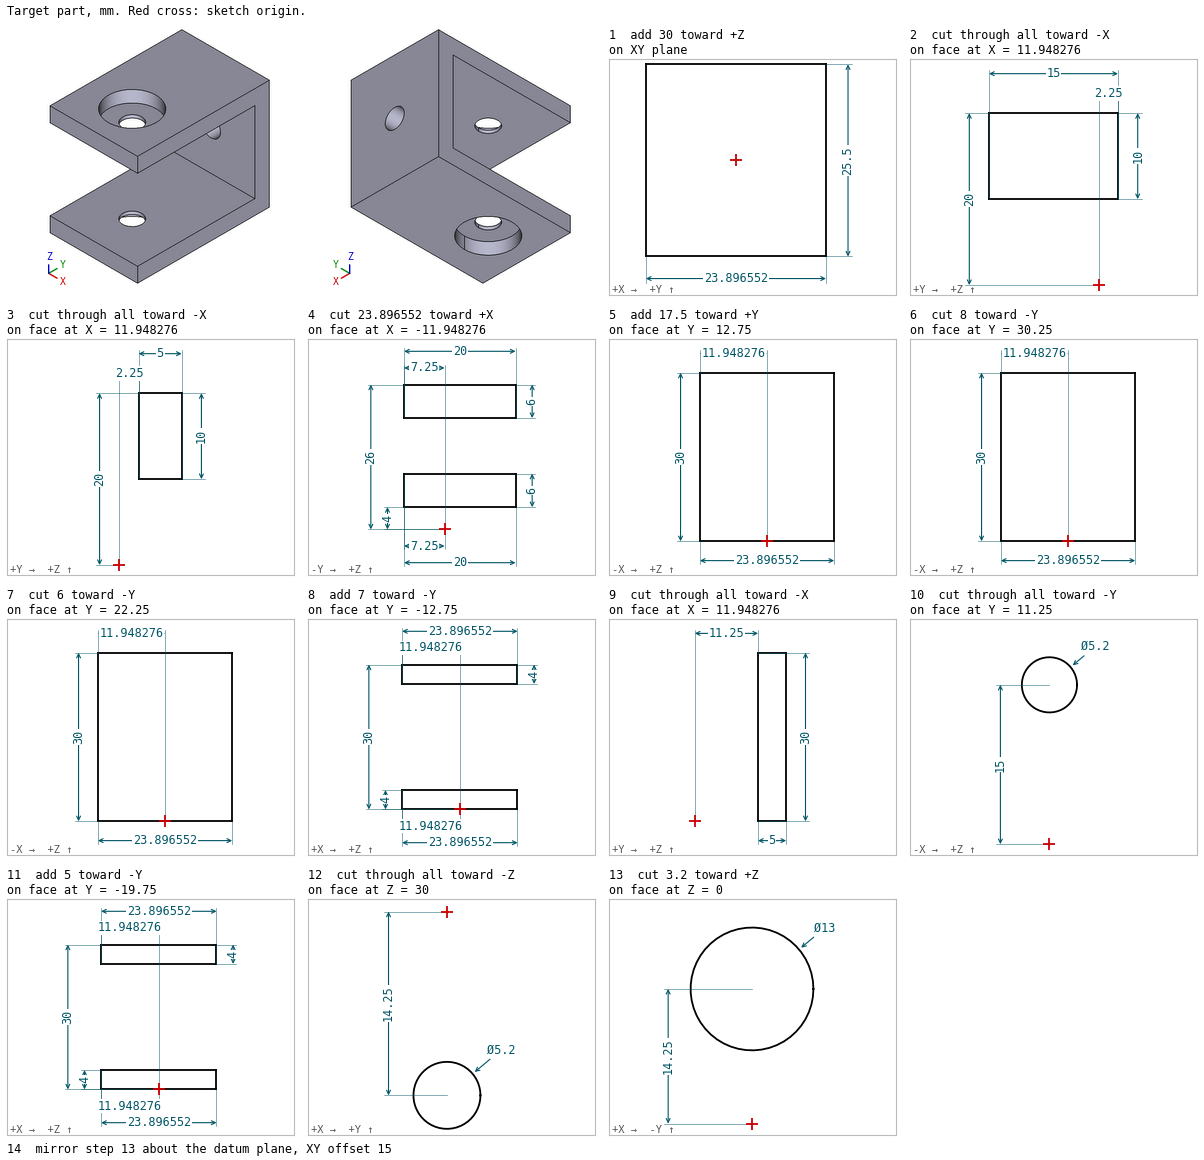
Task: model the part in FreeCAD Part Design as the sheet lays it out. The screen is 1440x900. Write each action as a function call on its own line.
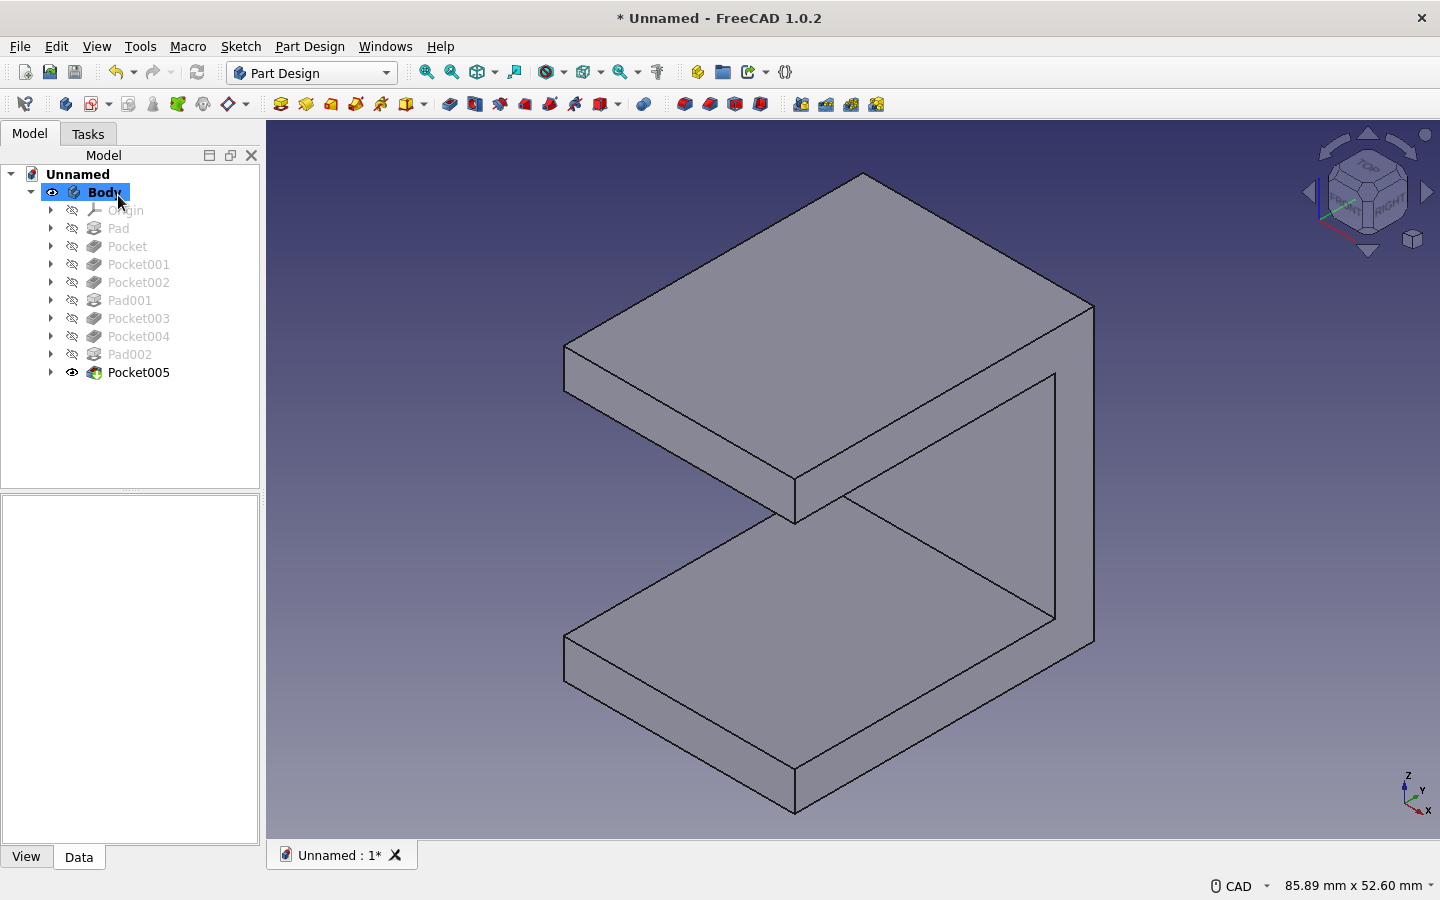
key(4)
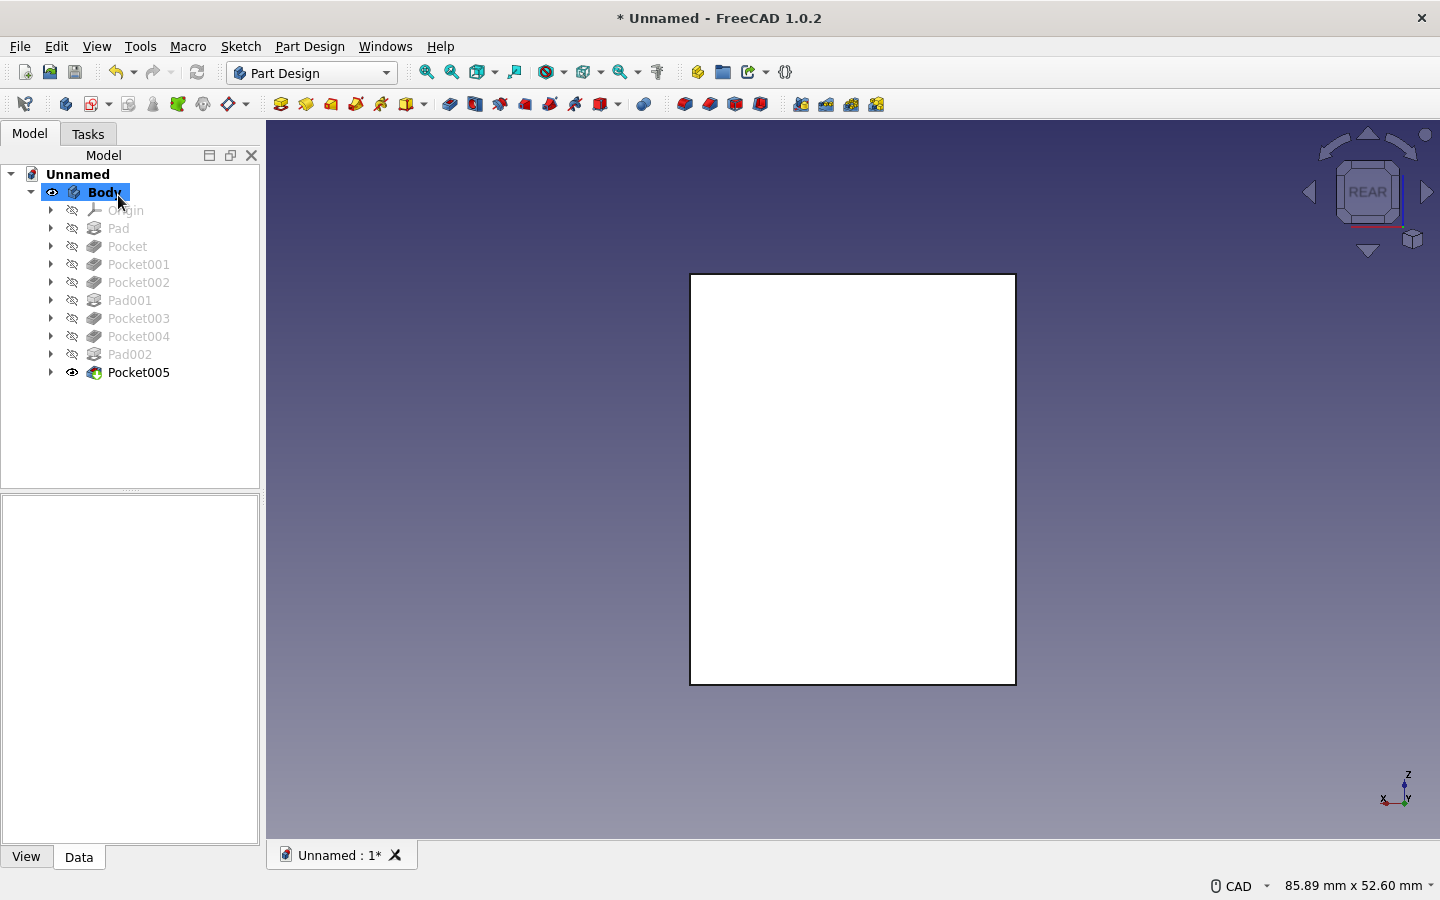
click(853, 479)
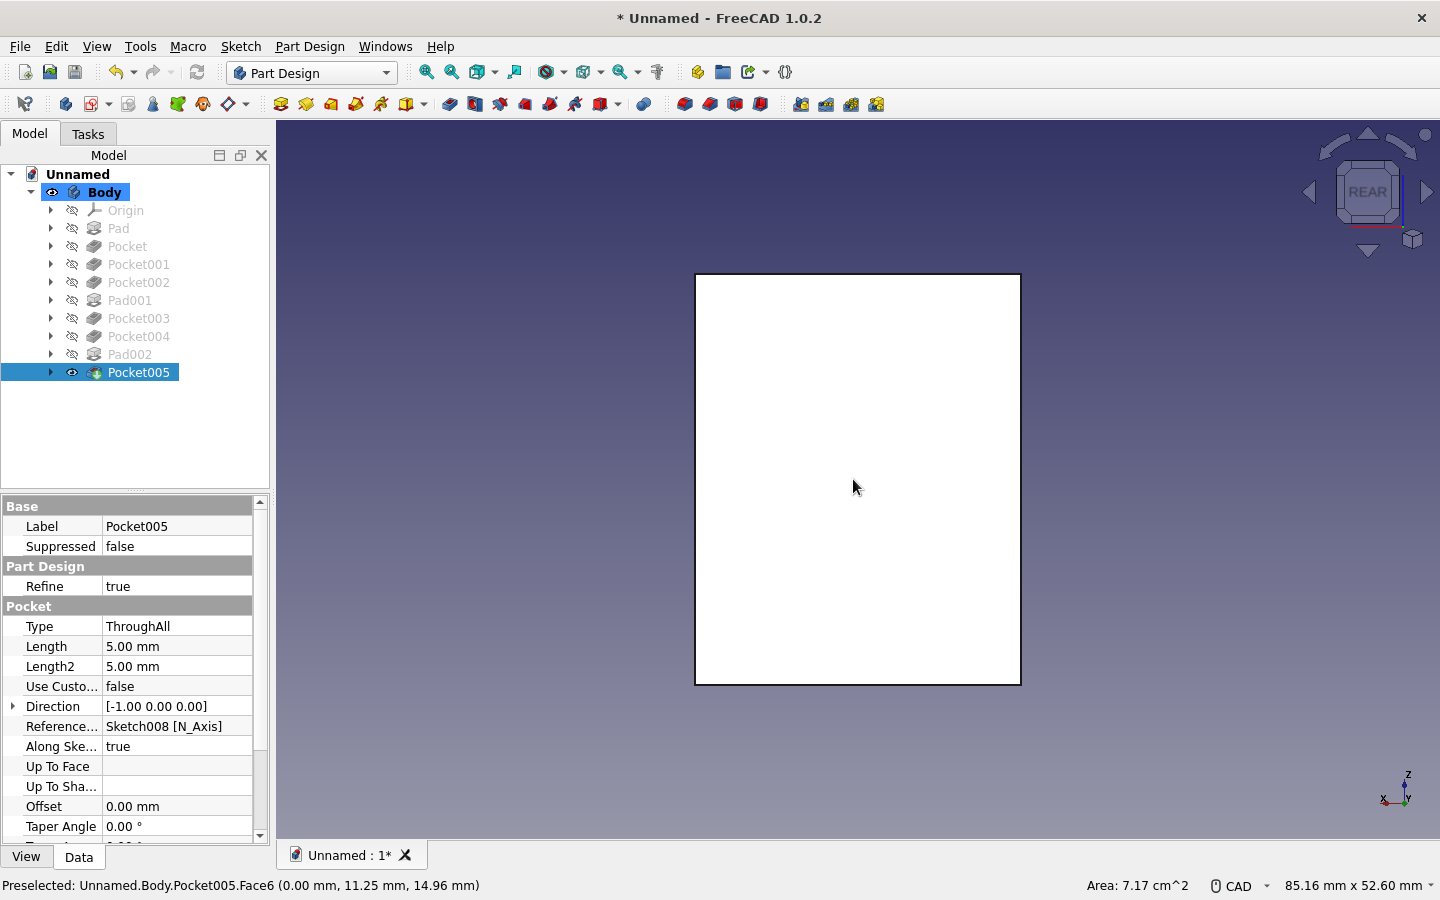
click(90, 104)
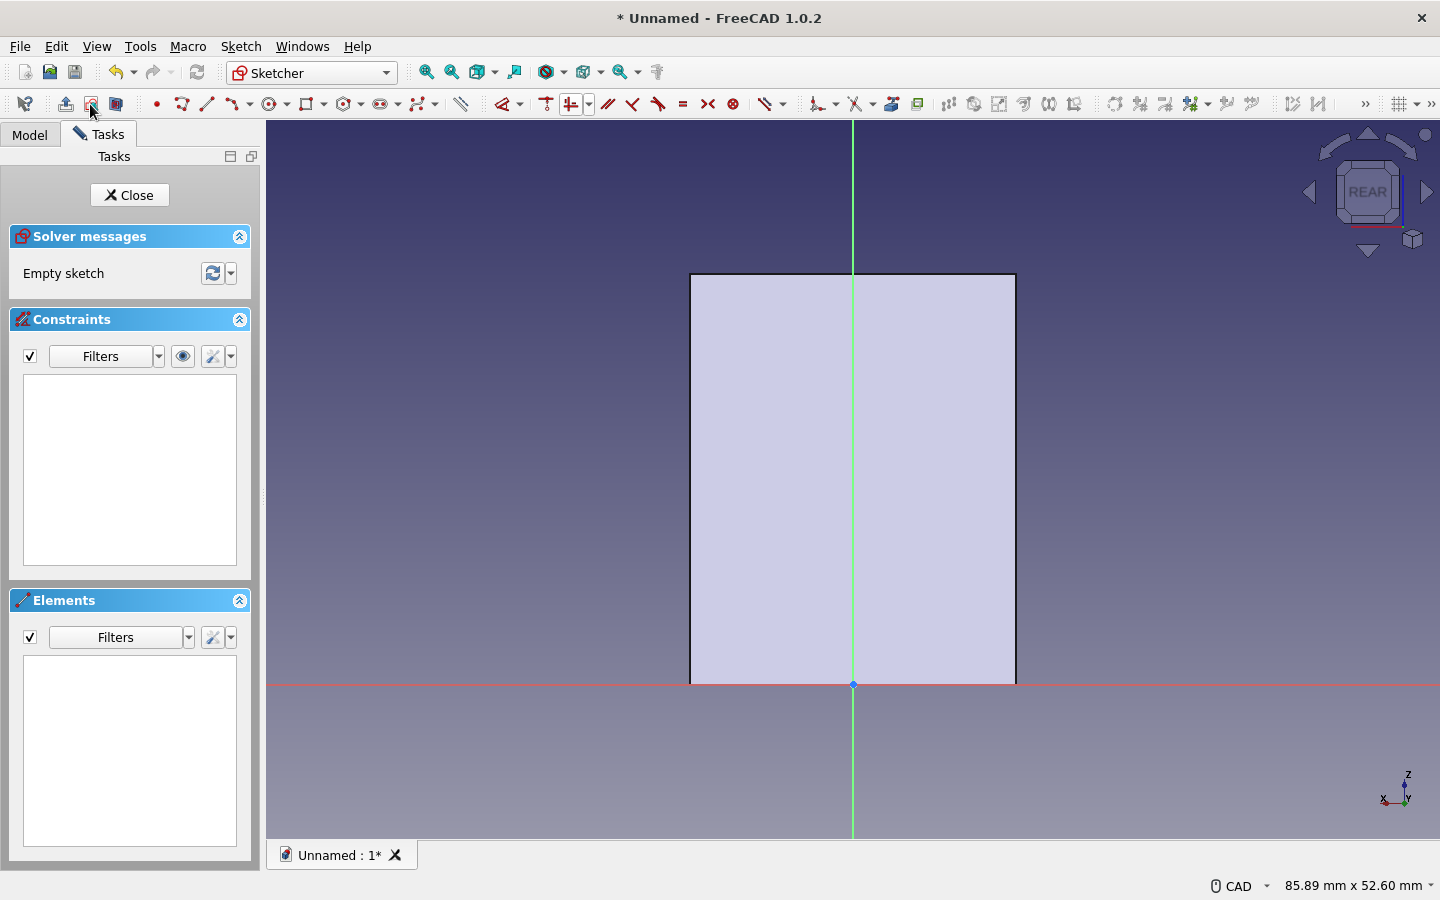
scroll(867, 480, up, 9)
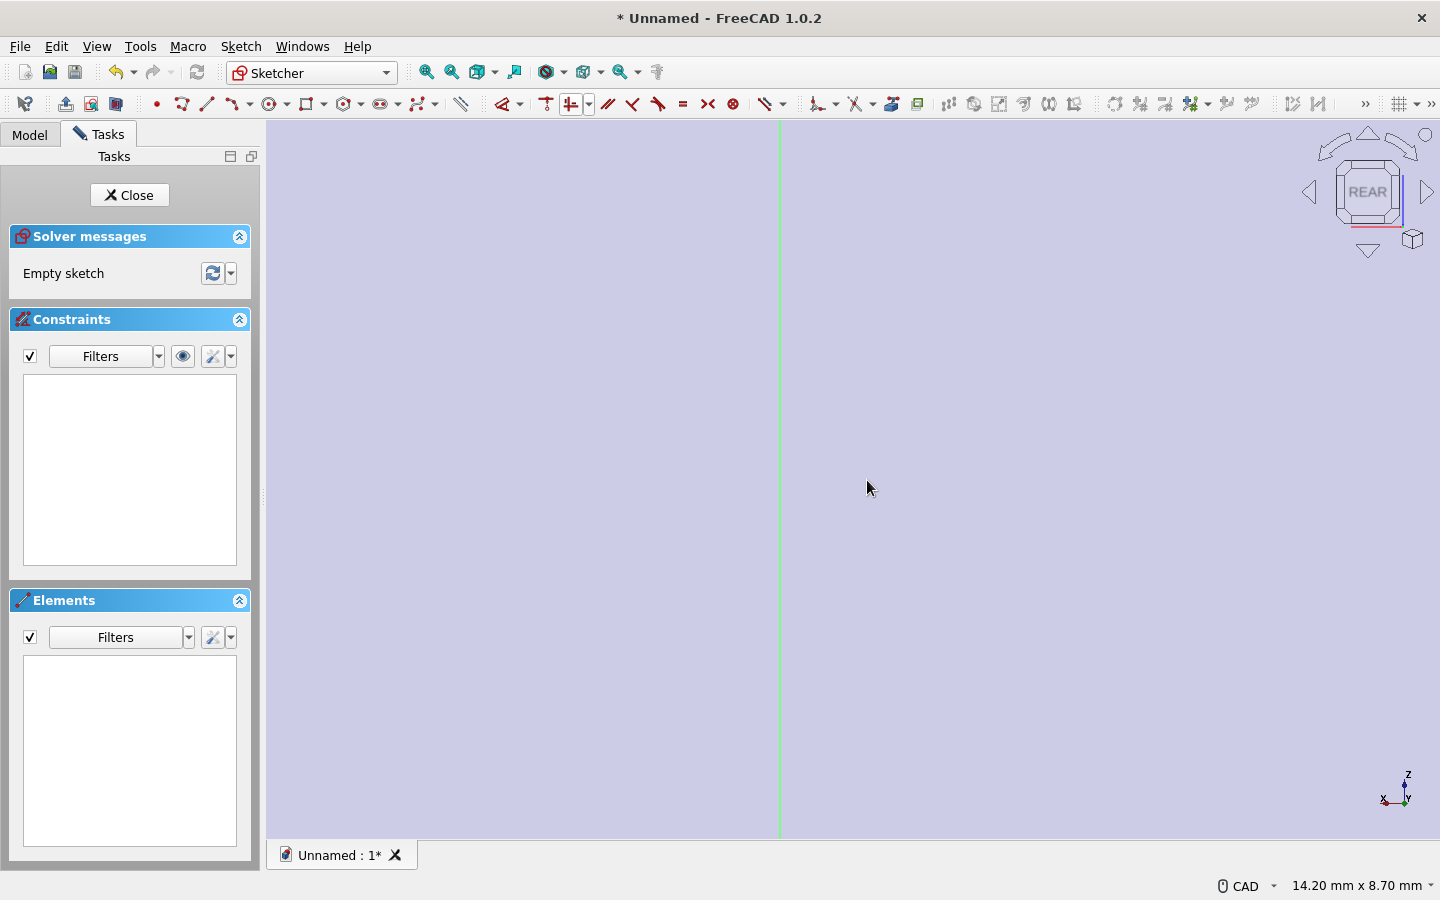
key(g)
key(c)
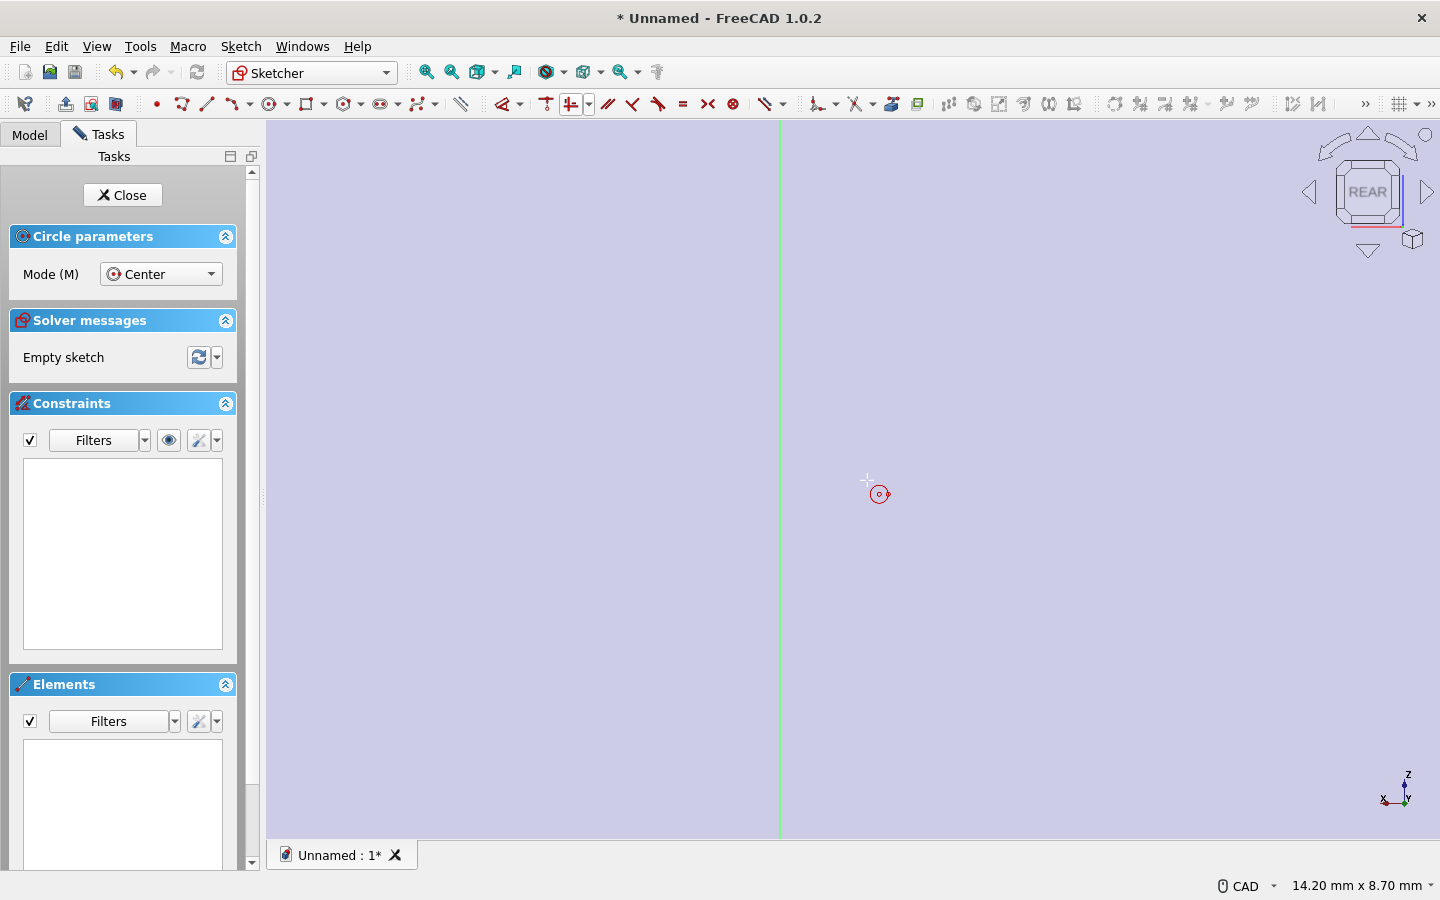
click(780, 474)
move(932, 322)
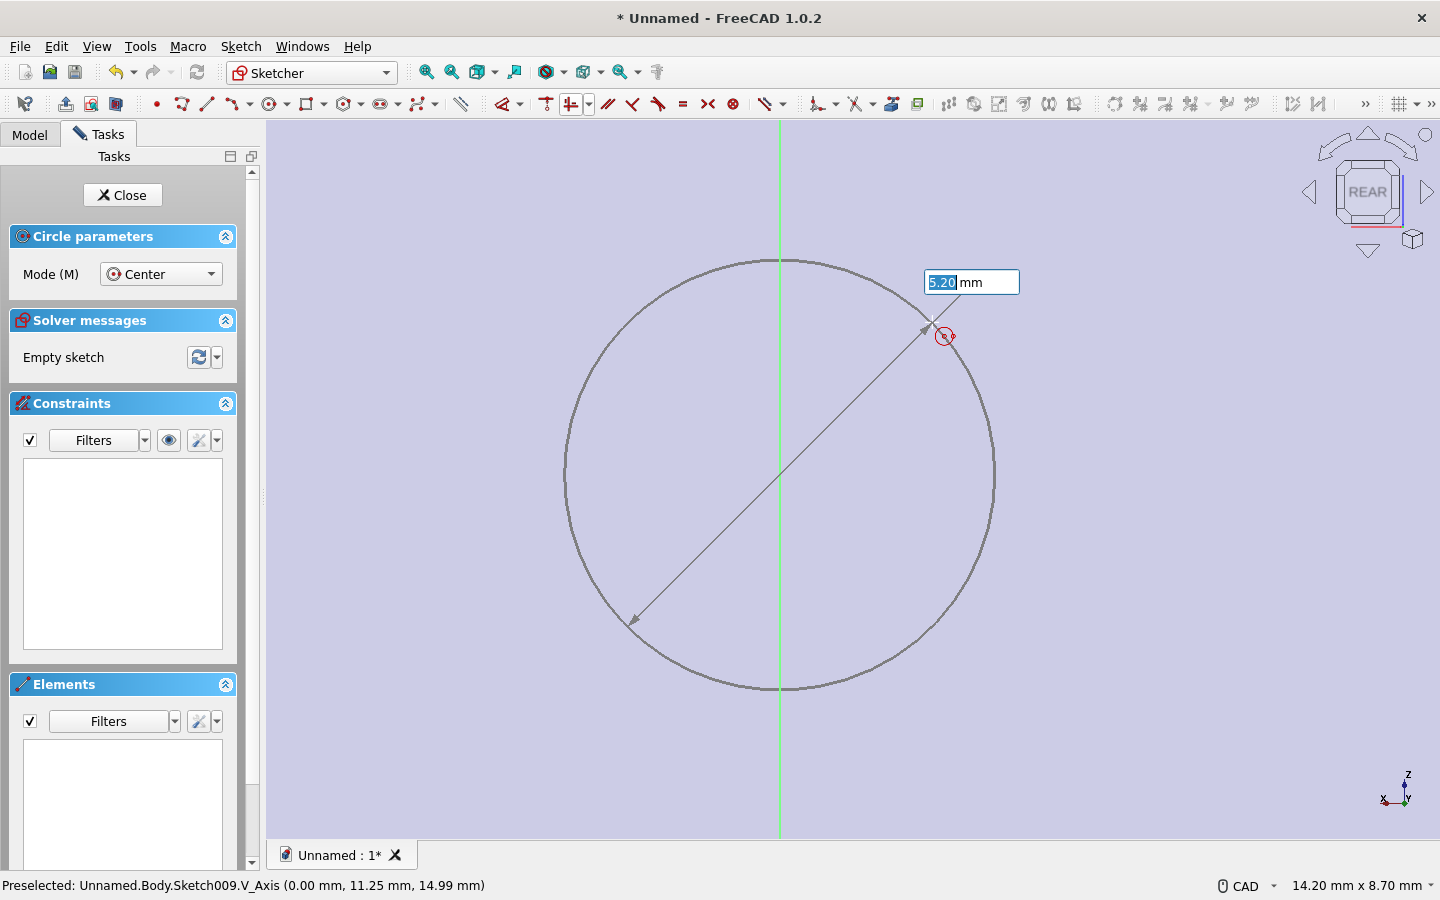
text(5.2)
key(Return)
key(Escape)